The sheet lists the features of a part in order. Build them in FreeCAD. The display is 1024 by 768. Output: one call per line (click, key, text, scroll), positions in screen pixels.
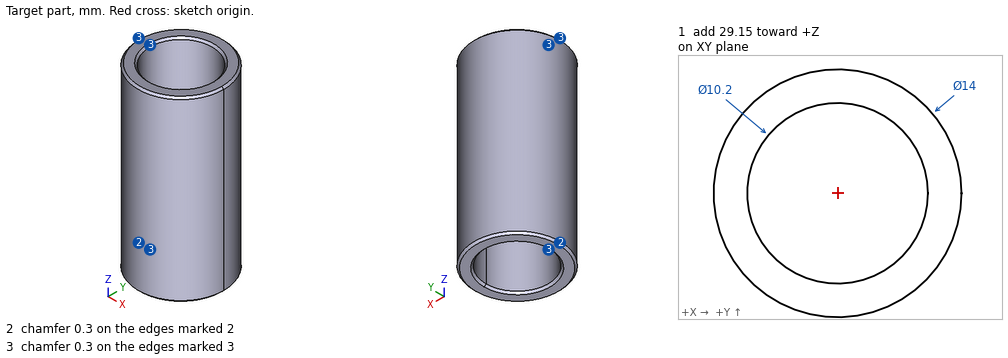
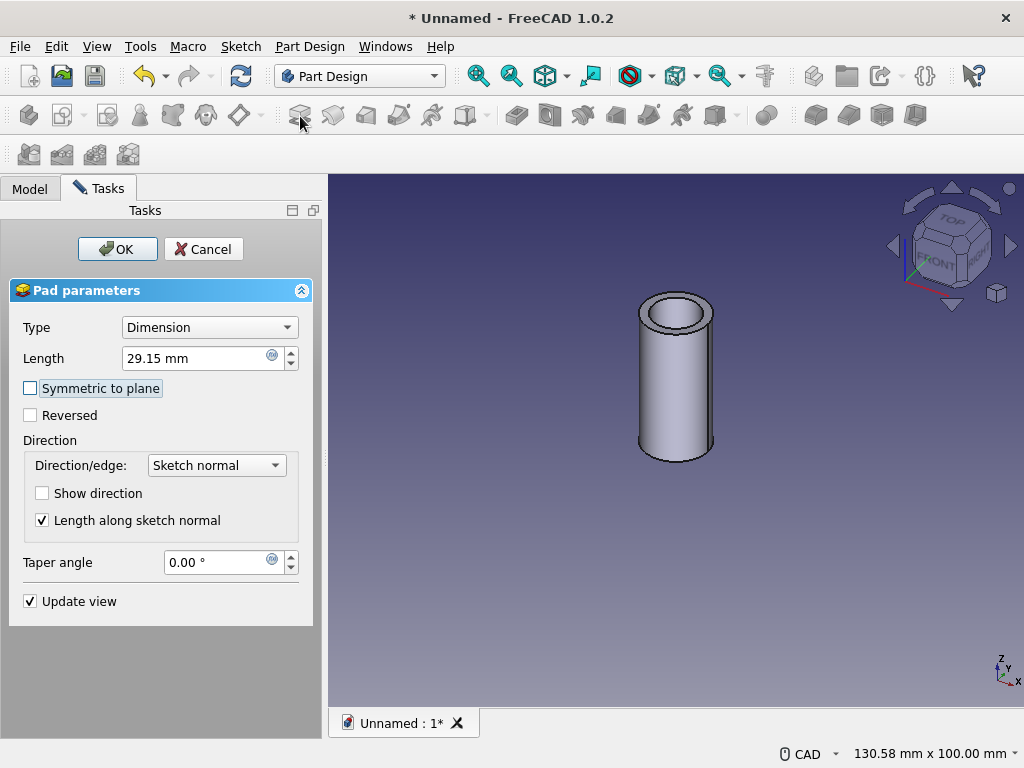
click(118, 249)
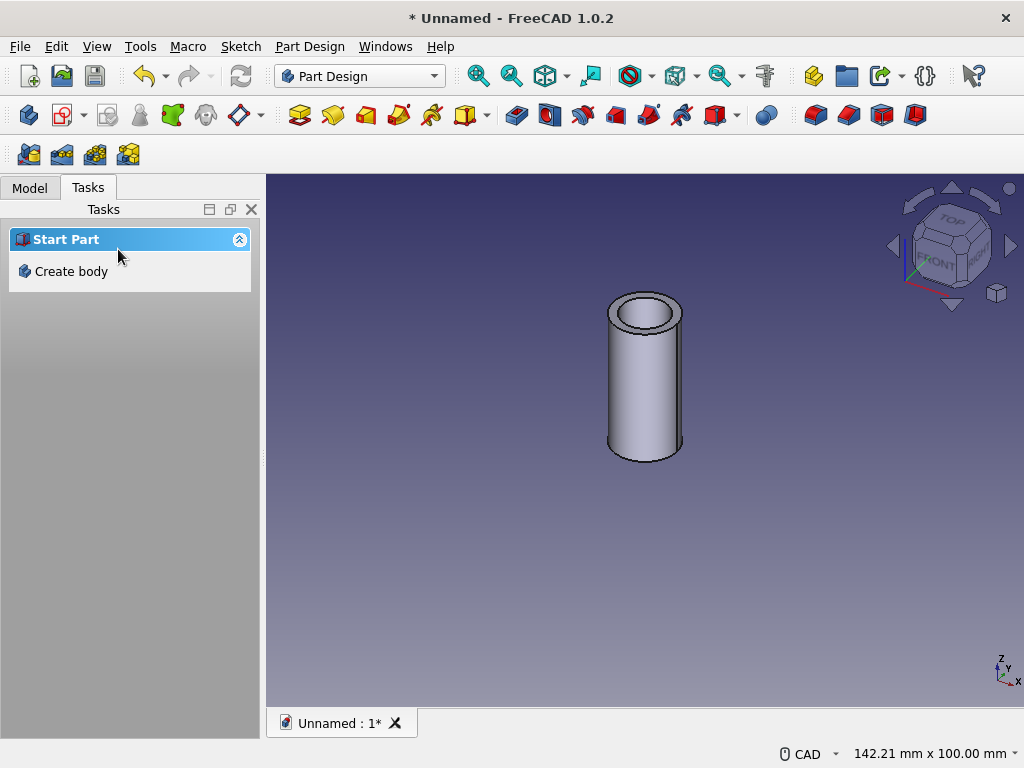
click(479, 76)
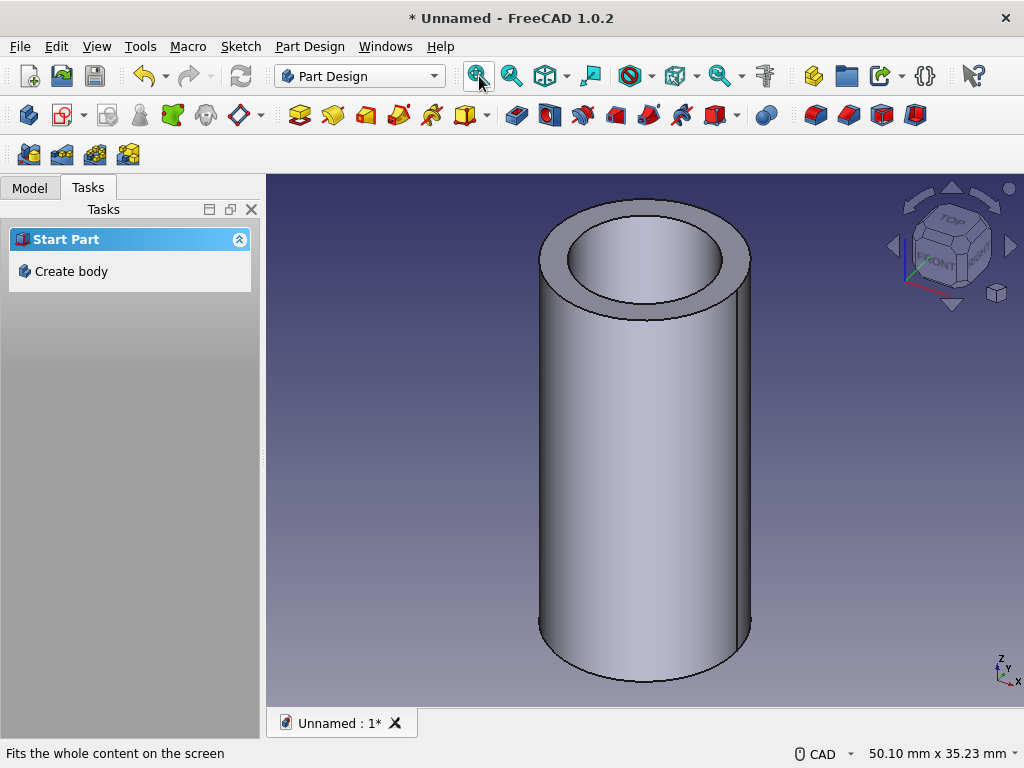
click(745, 640)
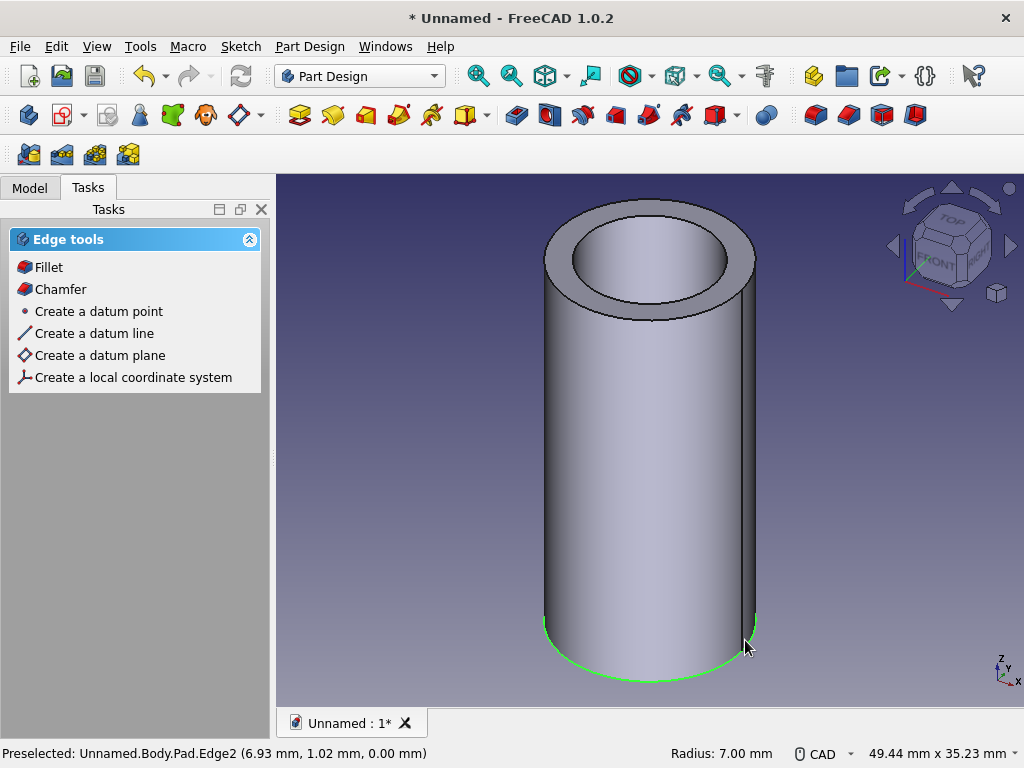
click(849, 116)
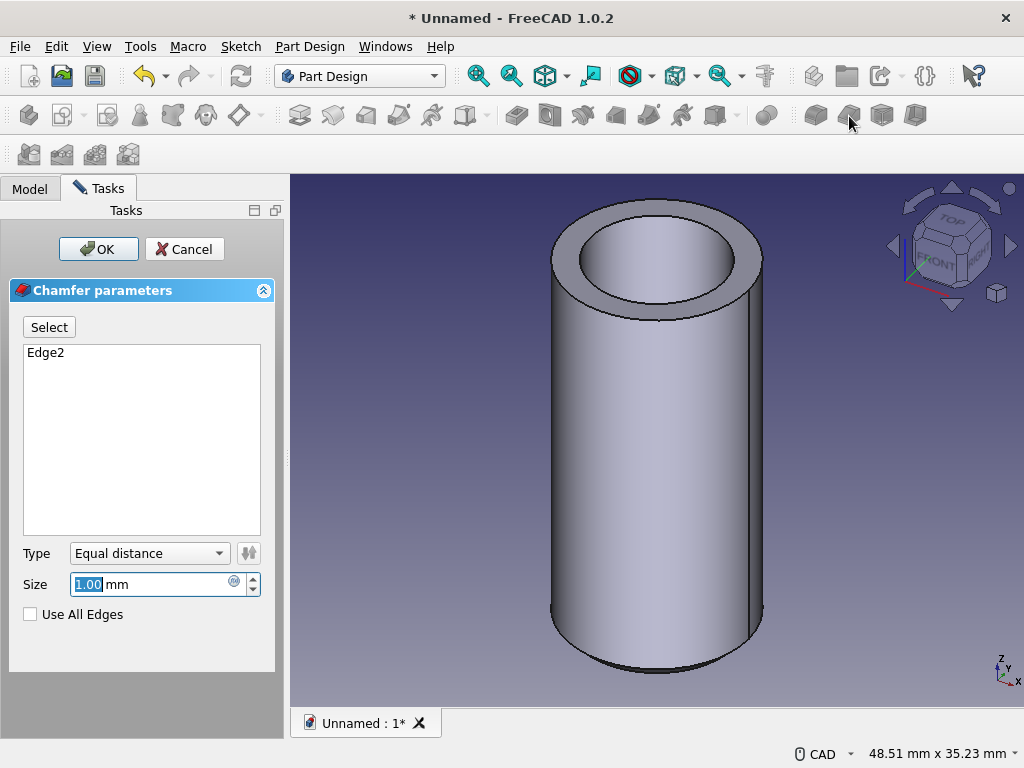
text(0.3)
key(Tab)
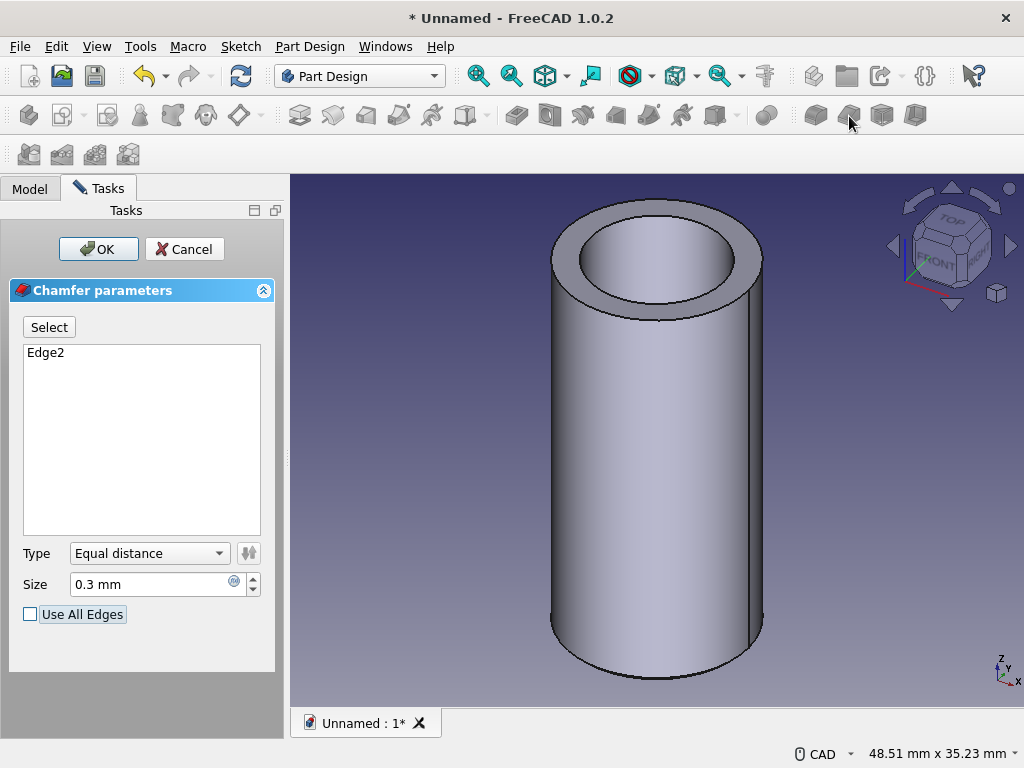
click(99, 249)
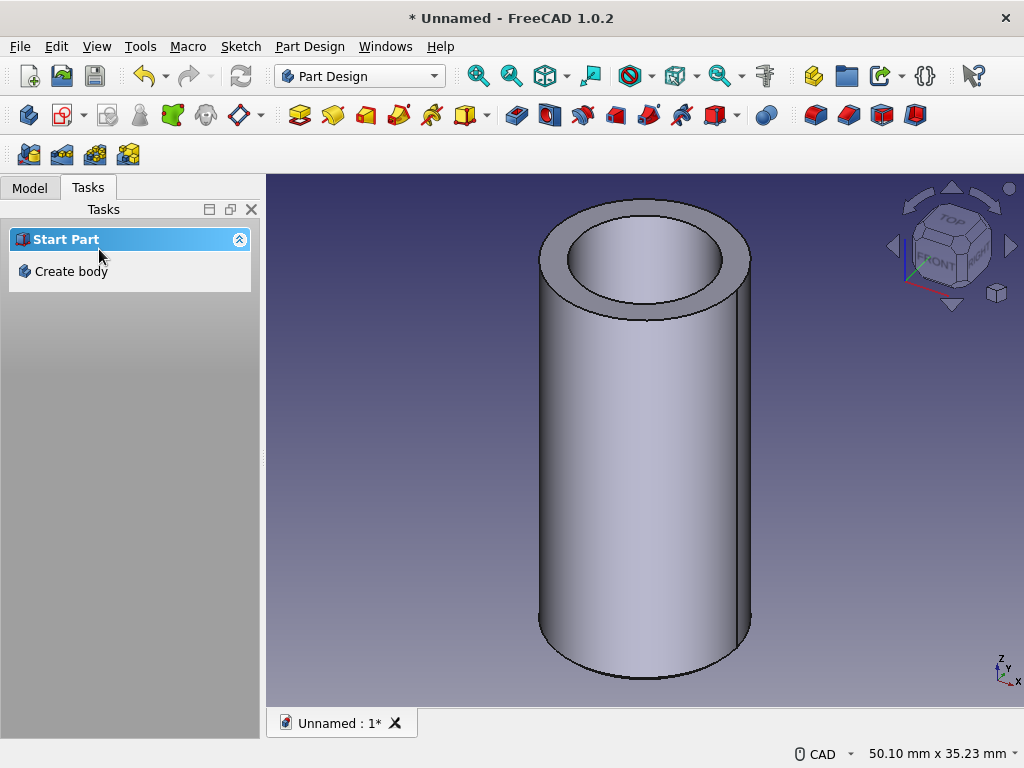
click(540, 265)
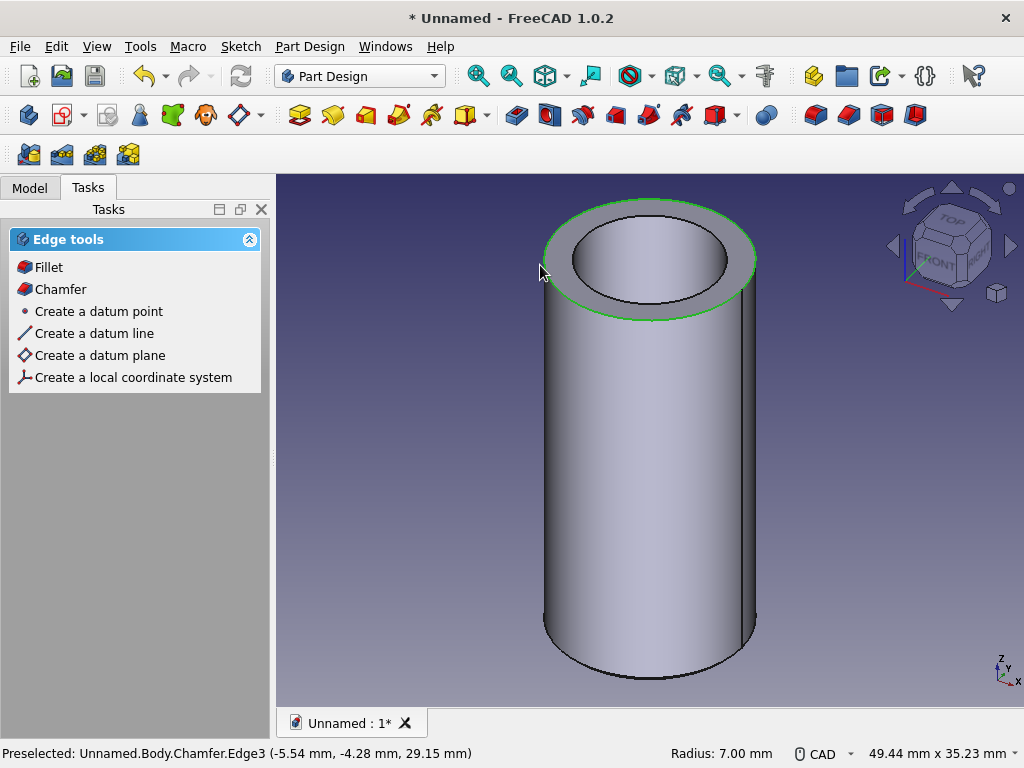
click(583, 237, ctrl)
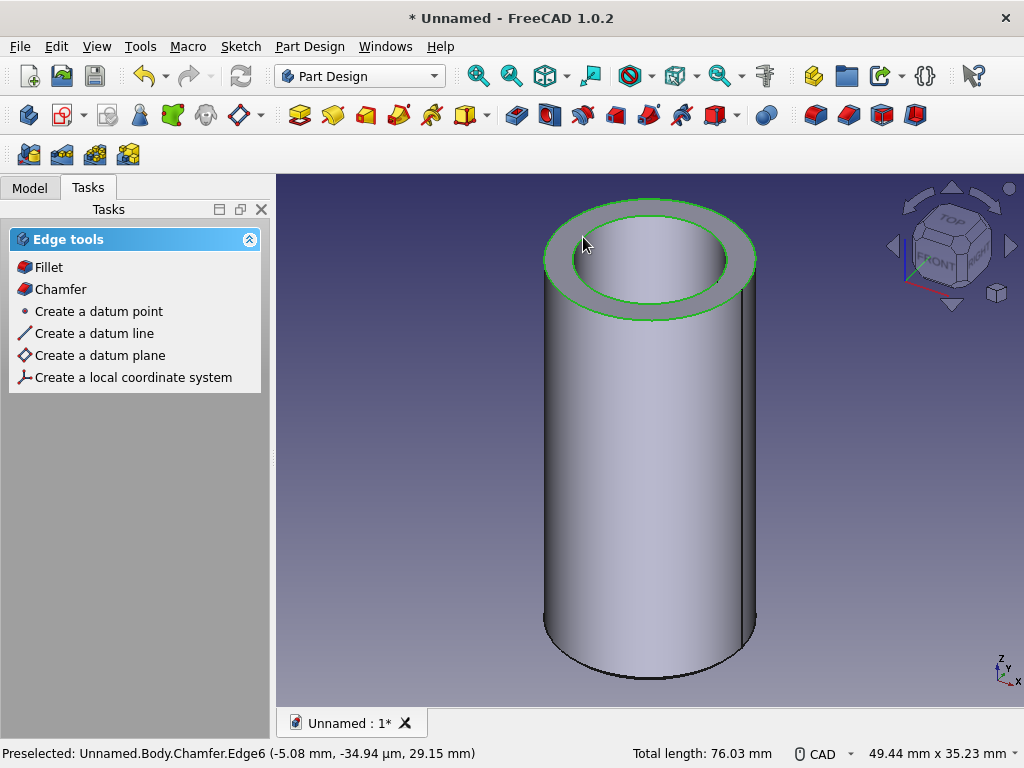
key(0)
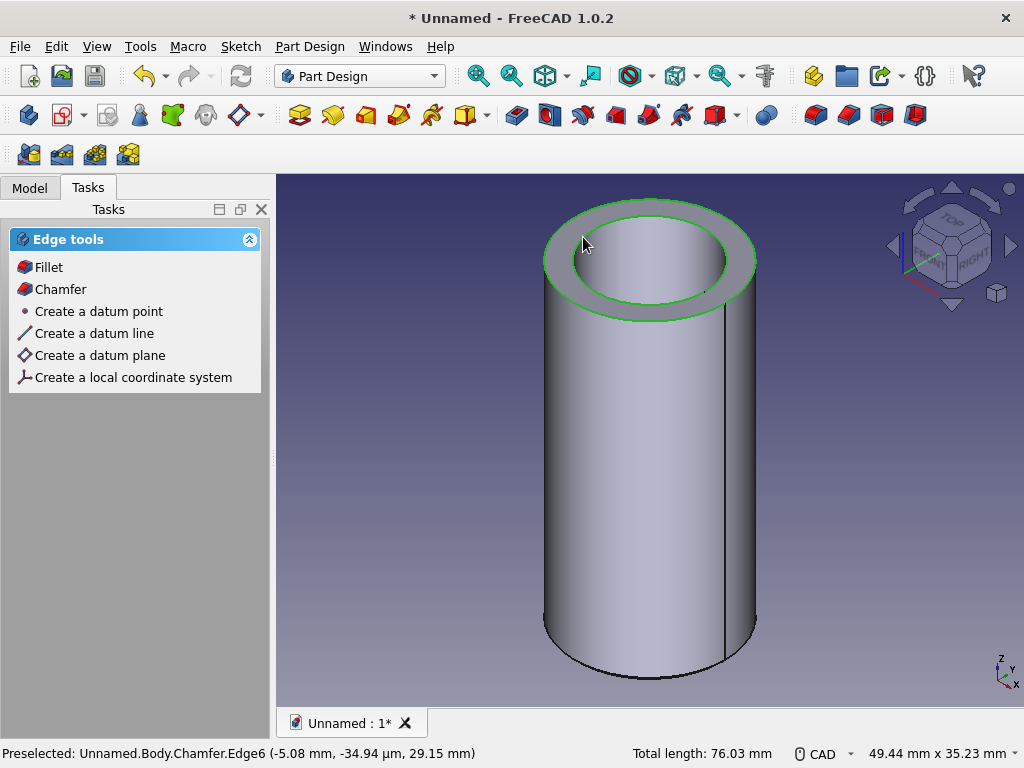
click(479, 76)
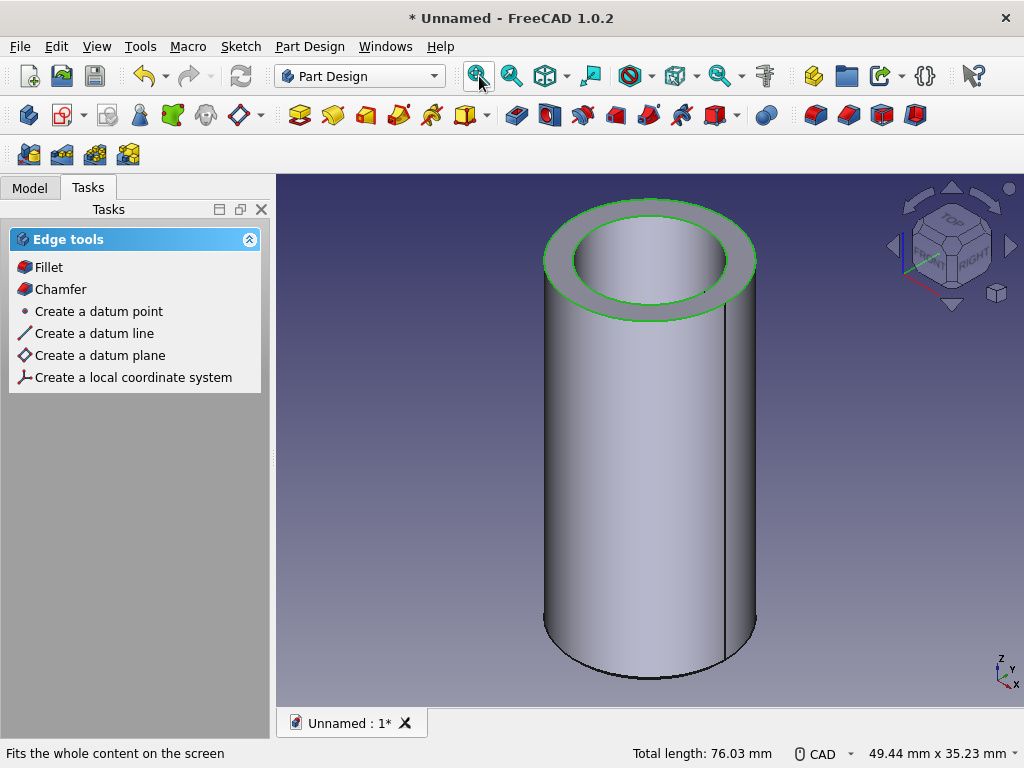
key(2)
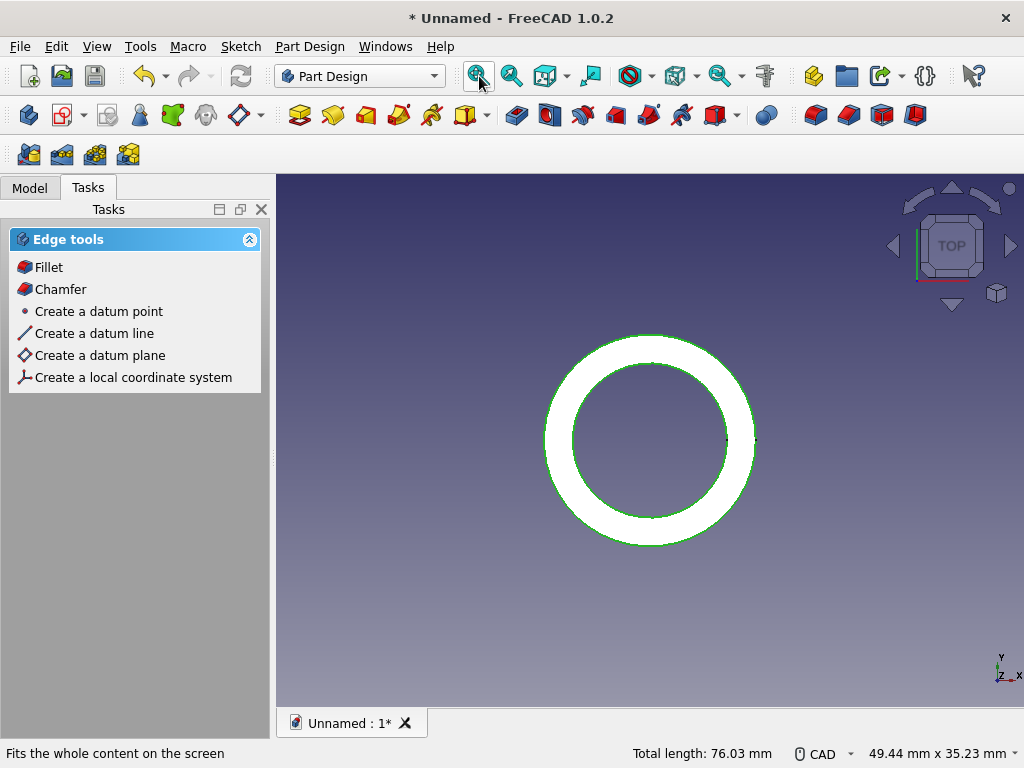
click(479, 76)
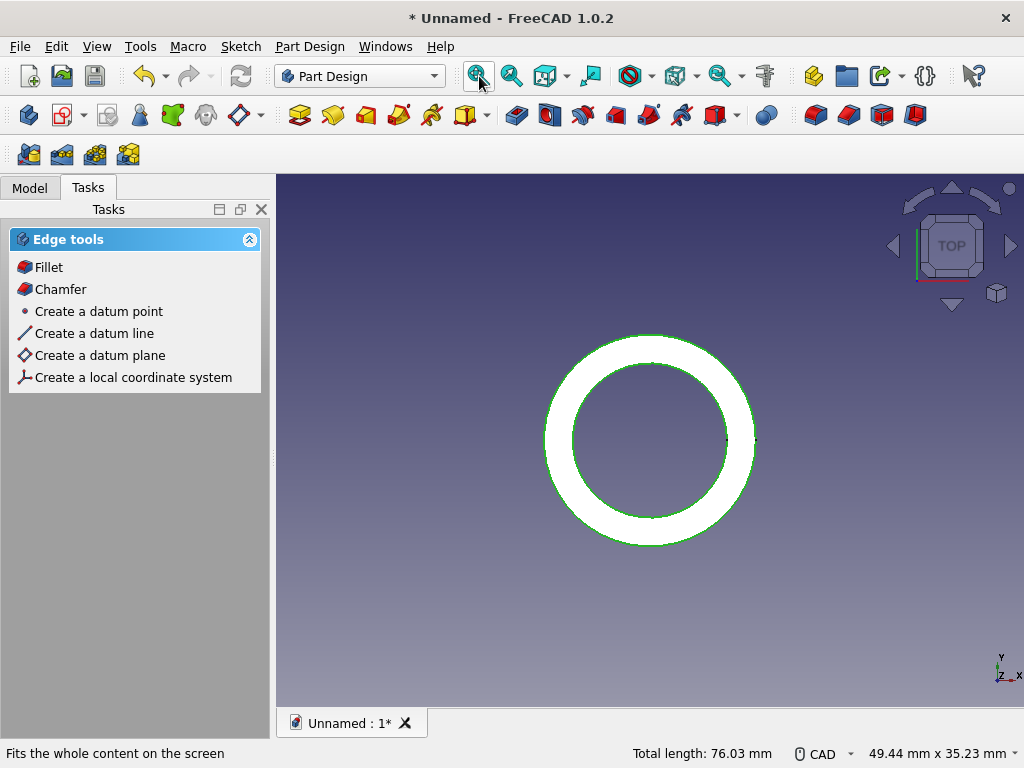
key(1)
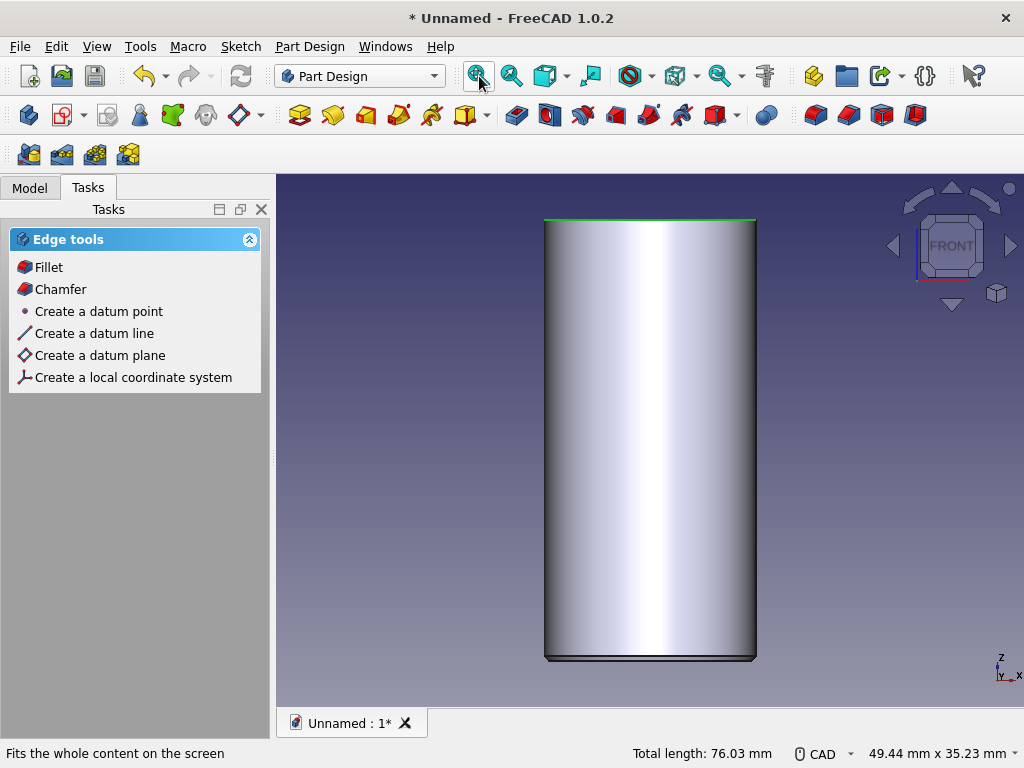
key(3)